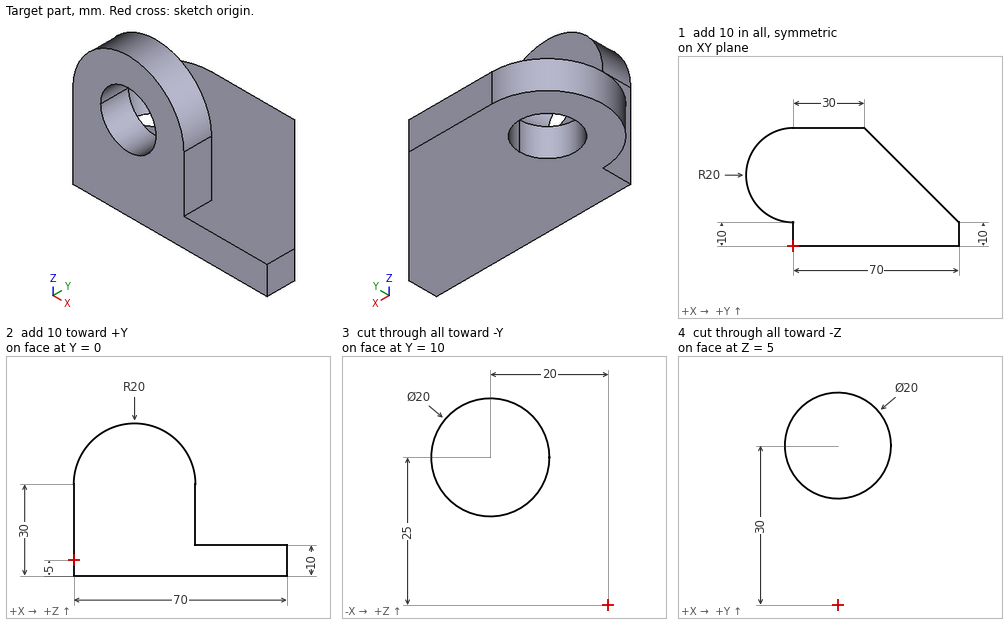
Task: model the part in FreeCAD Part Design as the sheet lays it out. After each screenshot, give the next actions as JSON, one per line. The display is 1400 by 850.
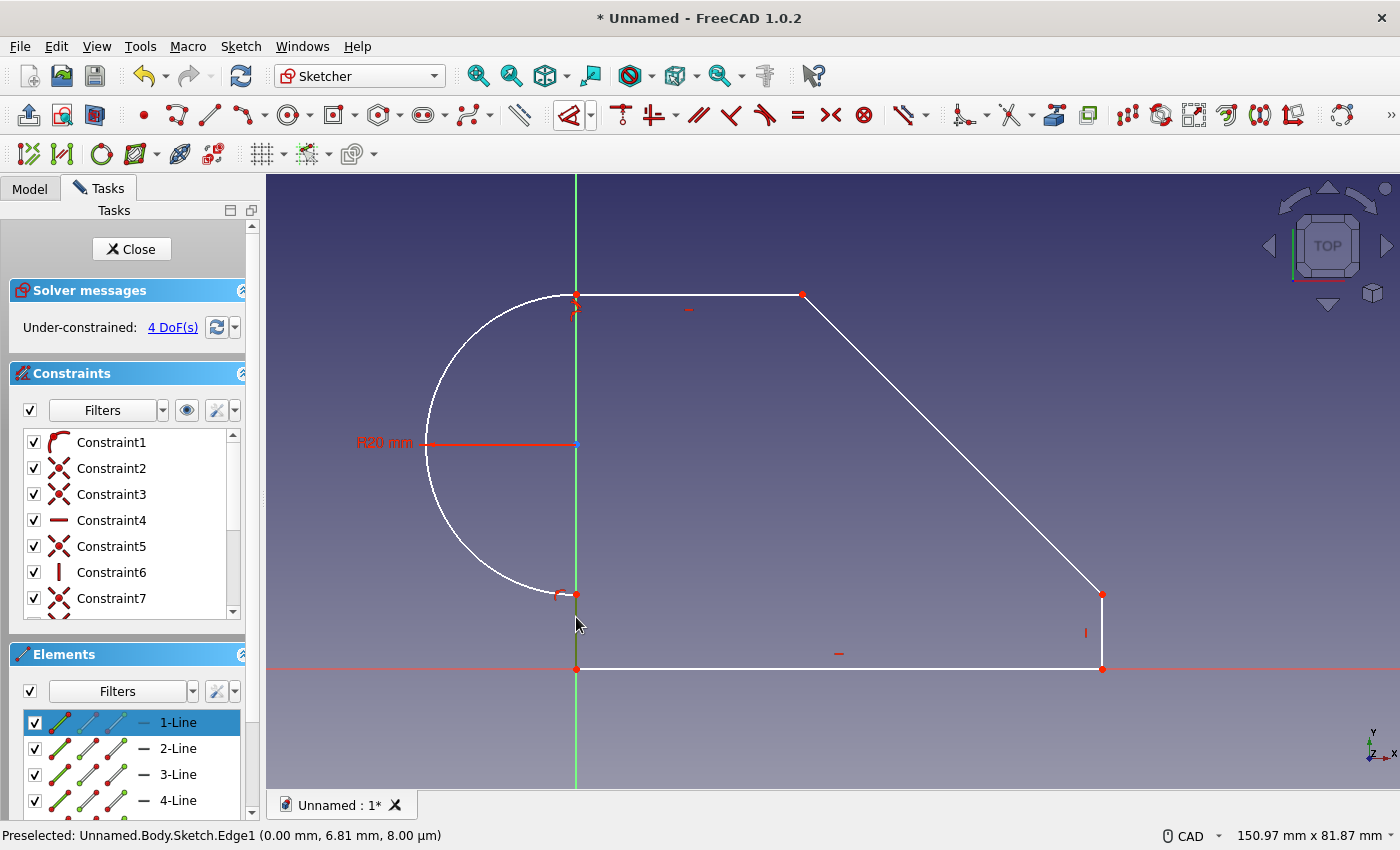
{"action": "left_click", "coordinate": [590, 116]}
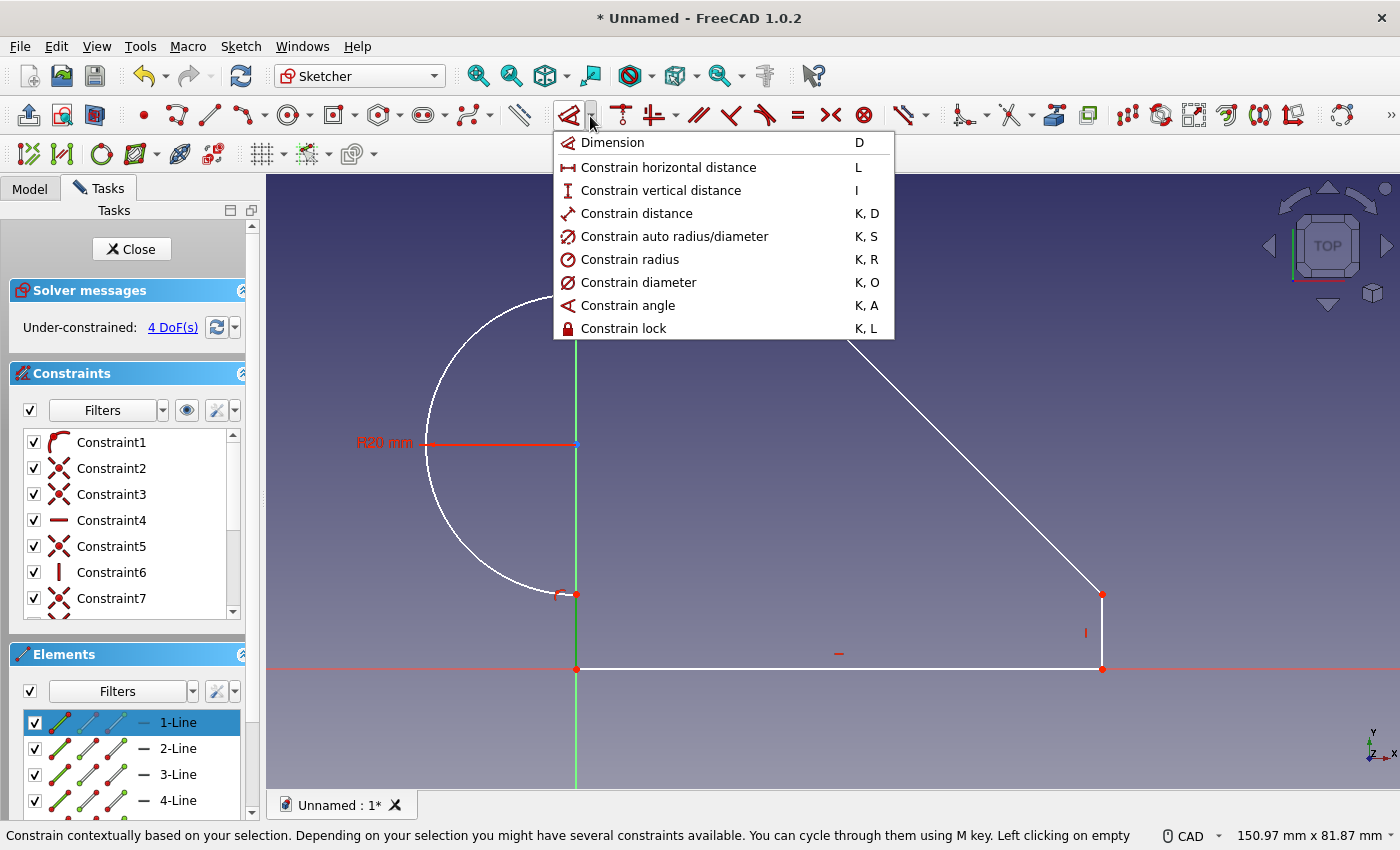
{"action": "left_click", "coordinate": [724, 190]}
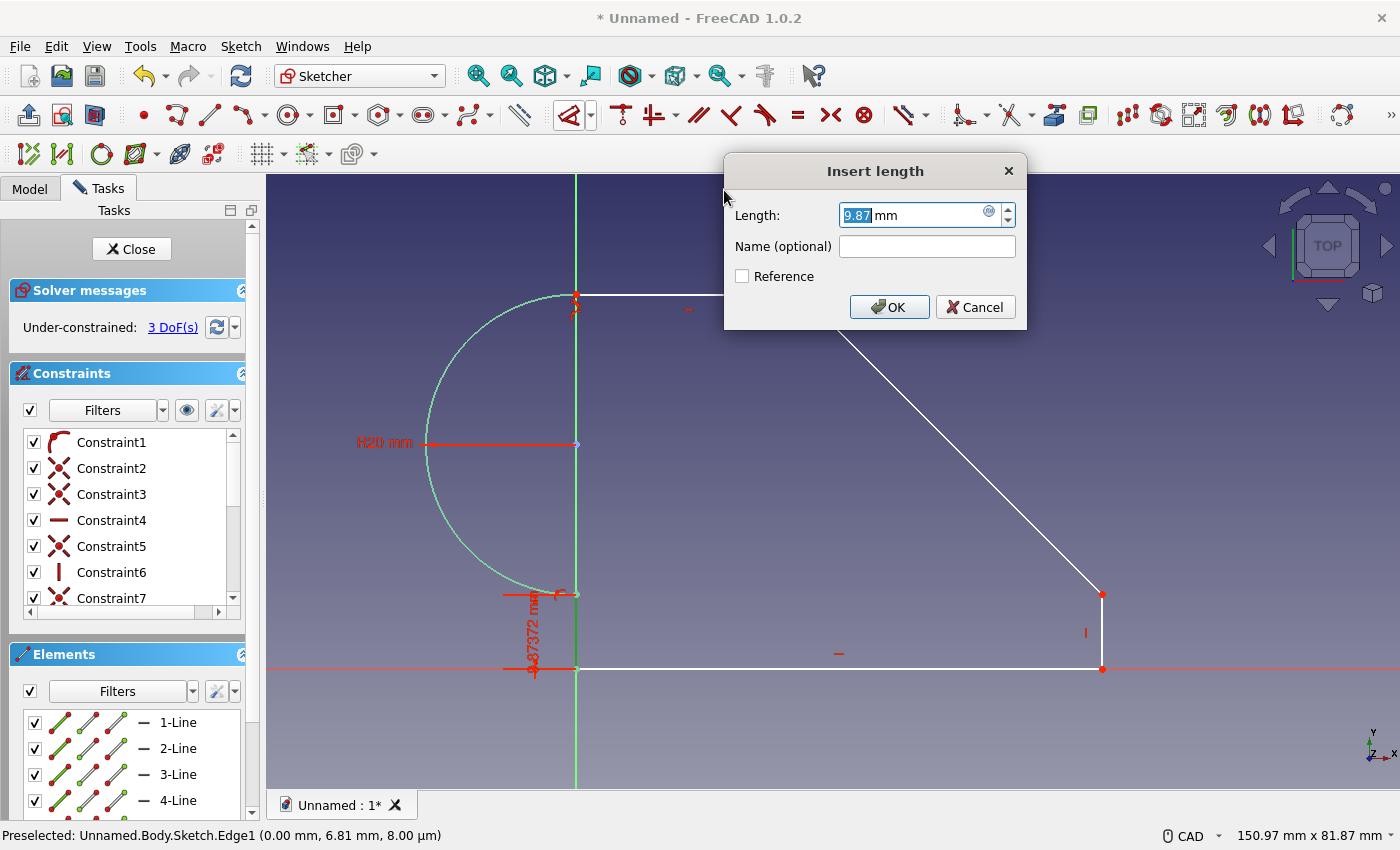
{"action": "type", "text": "10"}
{"action": "key", "text": "Return"}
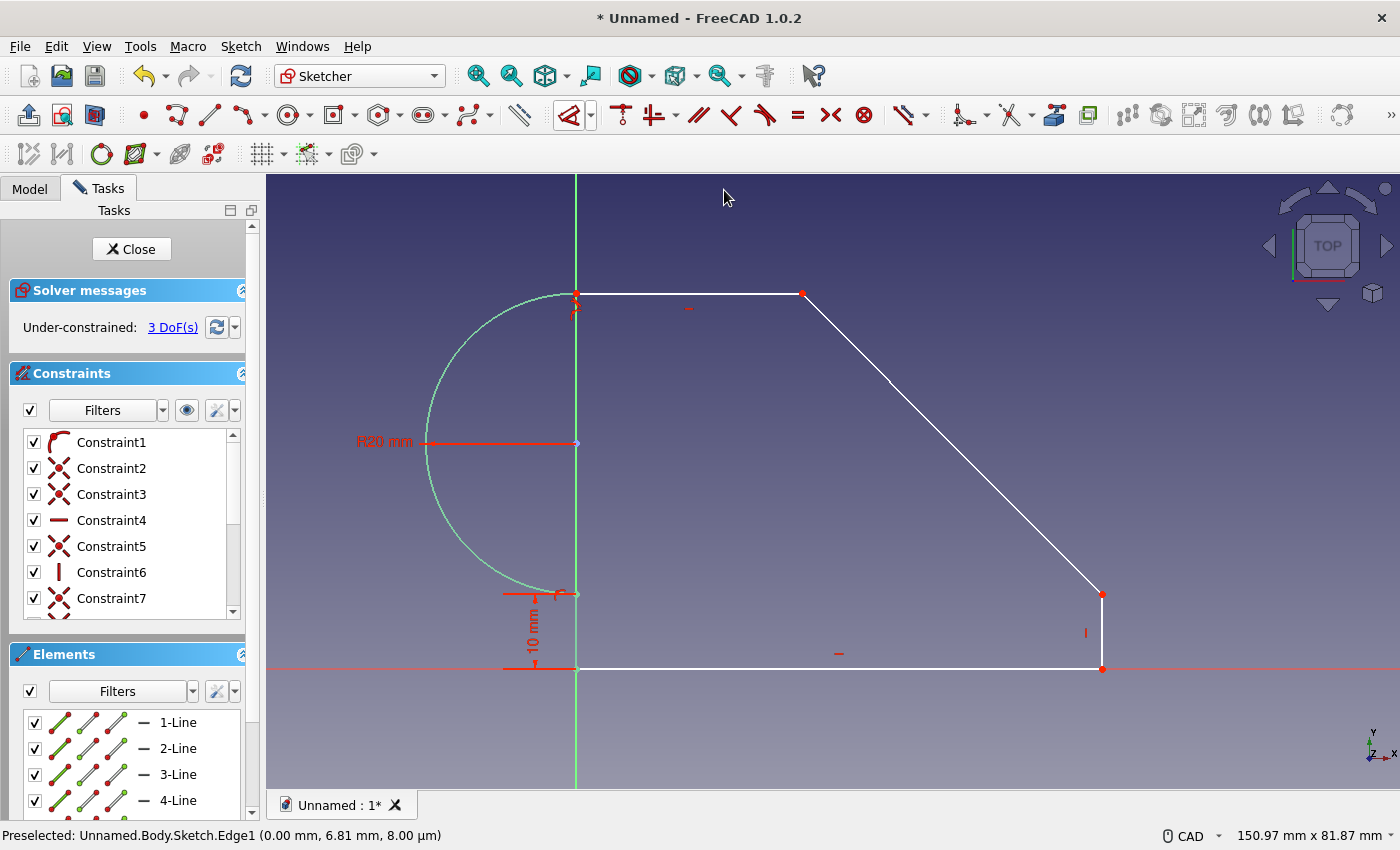
{"action": "left_click", "coordinate": [734, 669]}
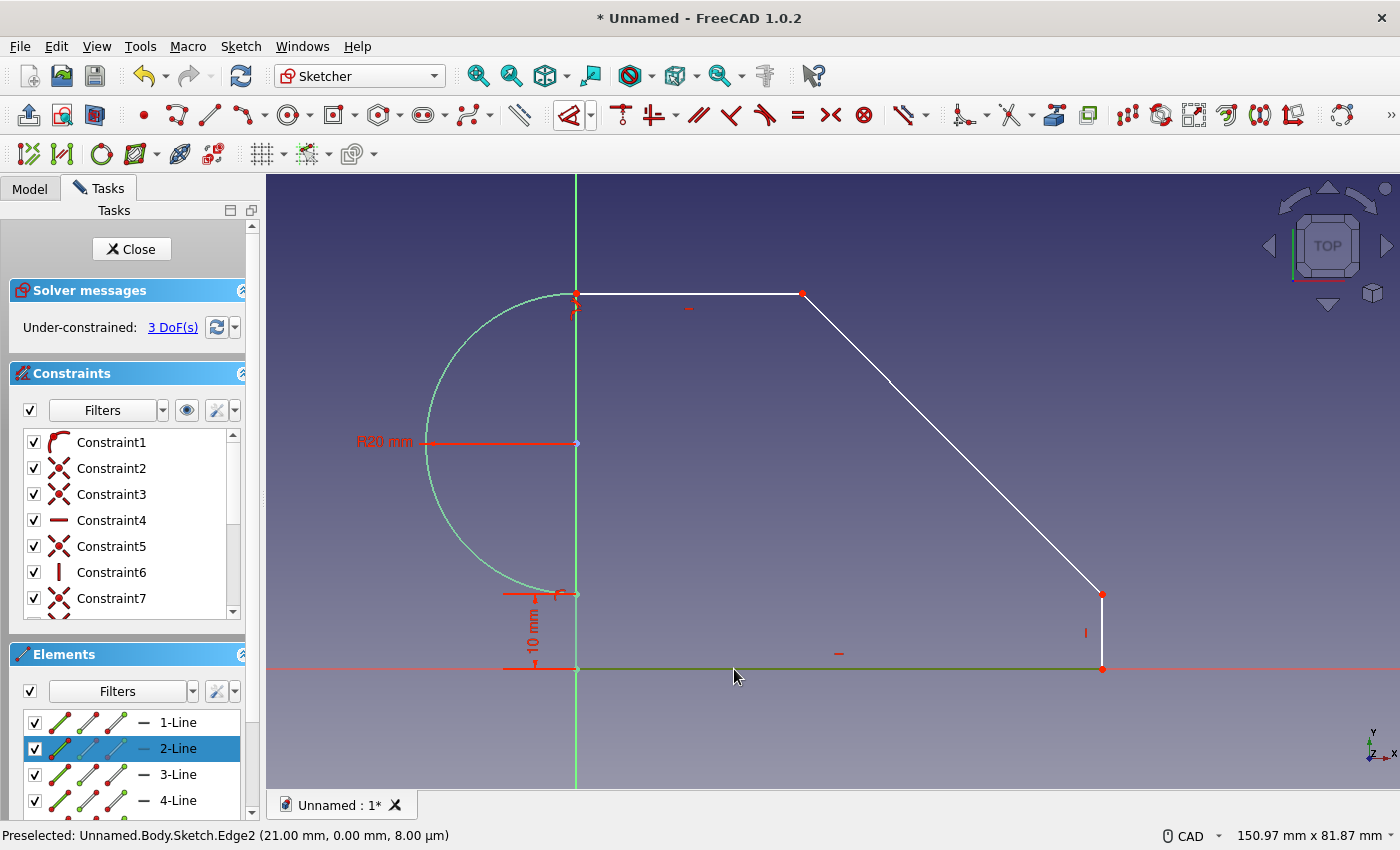
{"action": "left_click", "coordinate": [590, 116]}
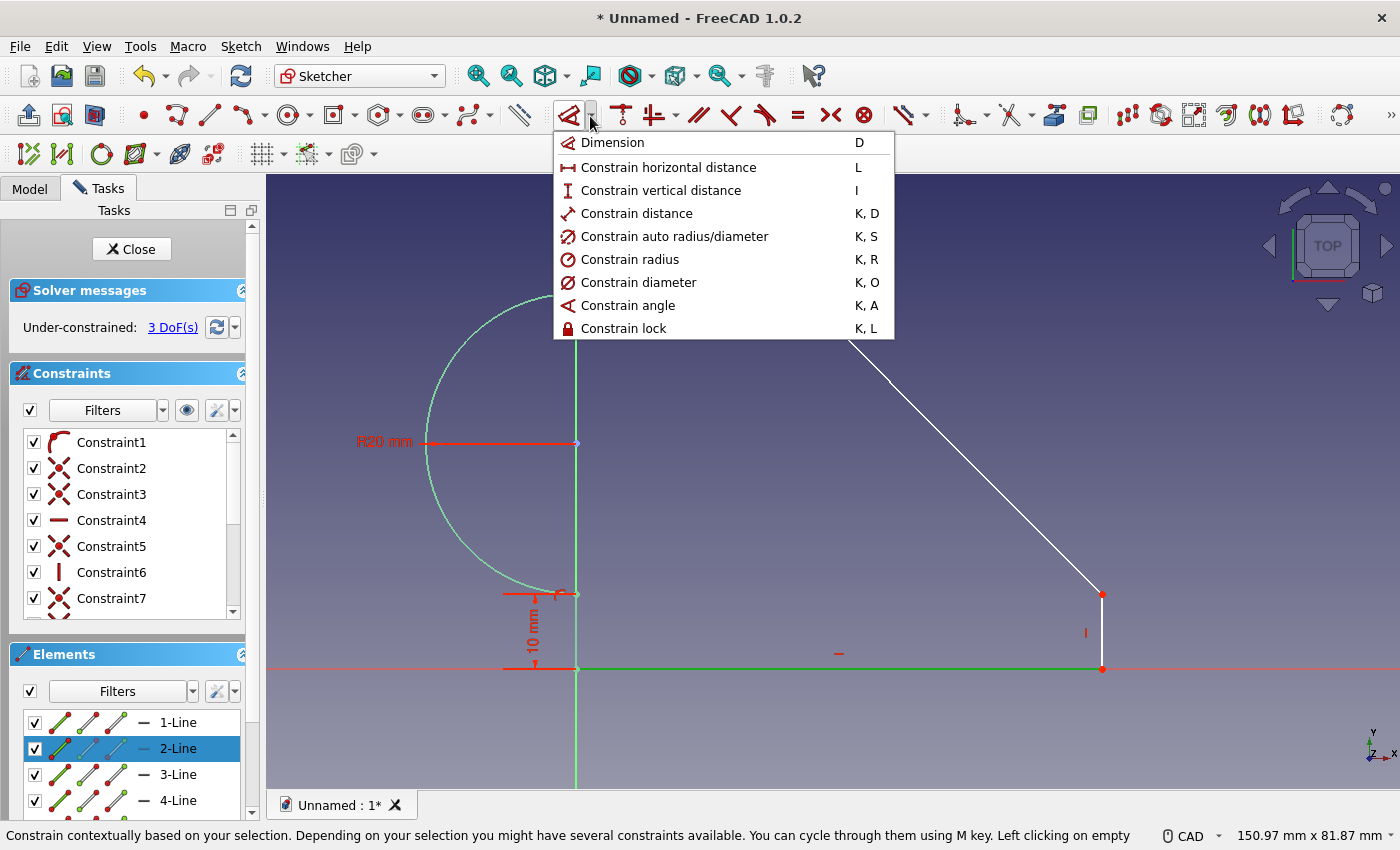
{"action": "left_click", "coordinate": [724, 168]}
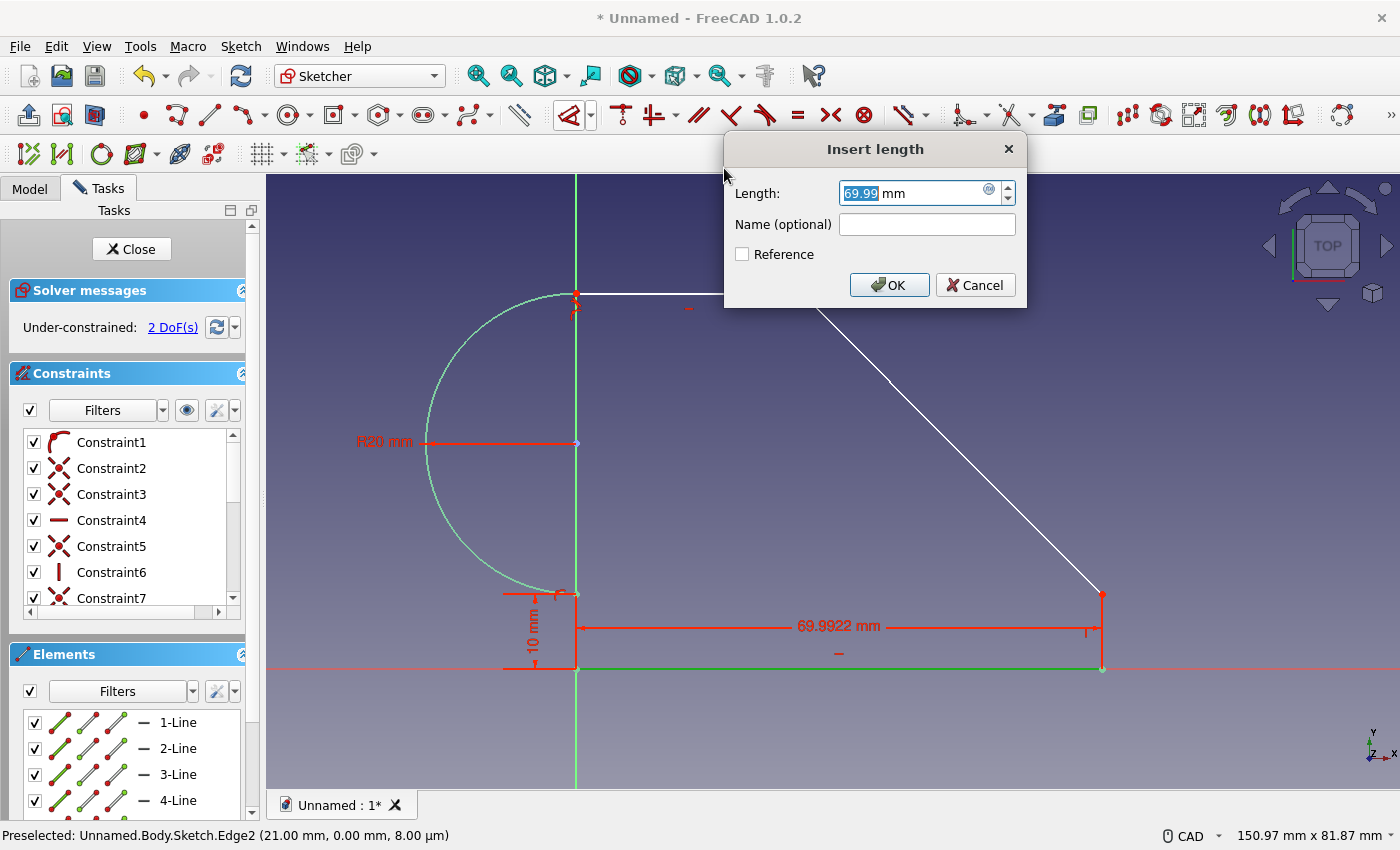
{"action": "type", "text": "70"}
{"action": "key", "text": "Return"}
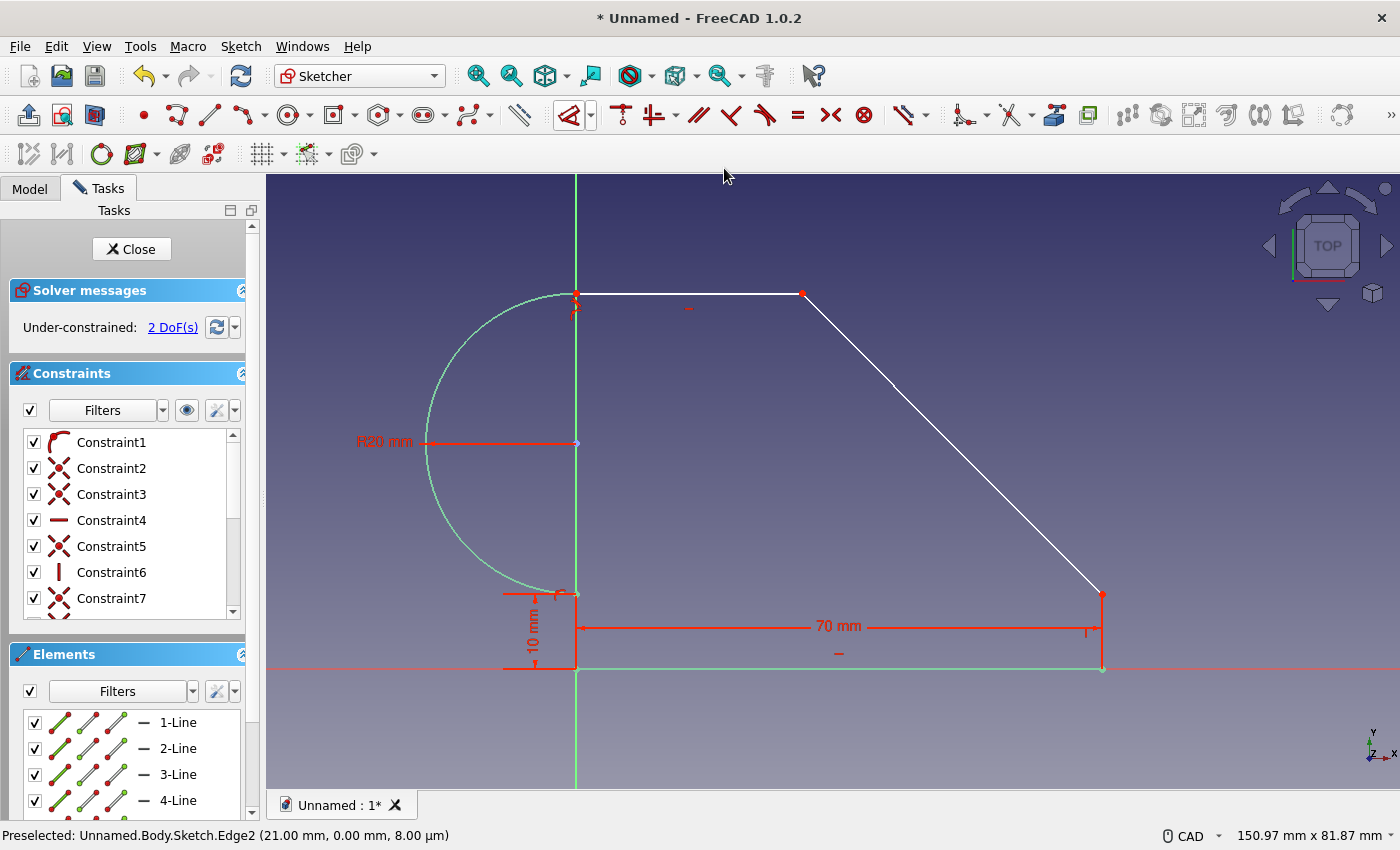
{"action": "left_click", "coordinate": [1102, 647]}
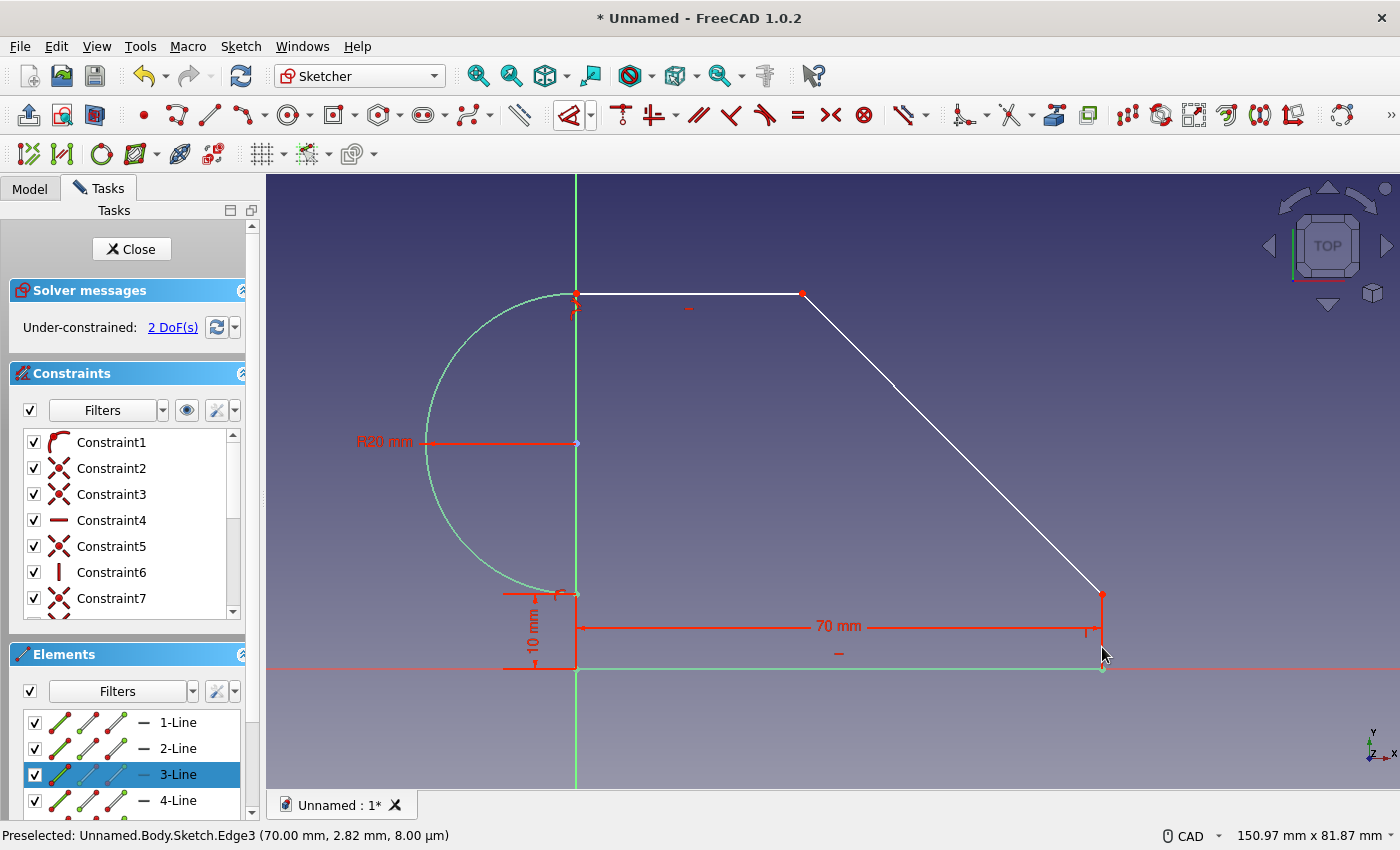
{"action": "key", "text": "i"}